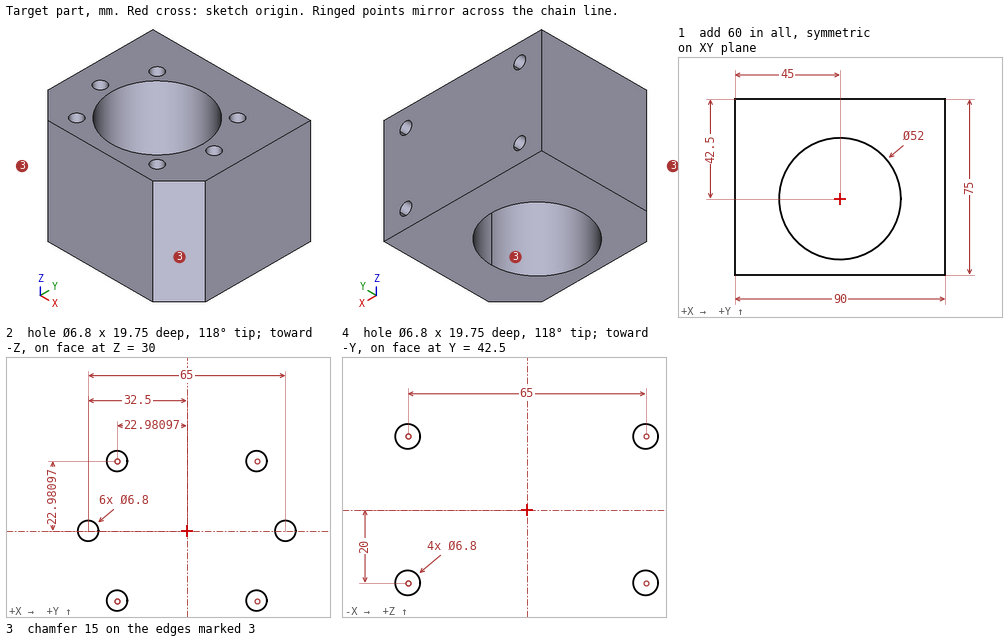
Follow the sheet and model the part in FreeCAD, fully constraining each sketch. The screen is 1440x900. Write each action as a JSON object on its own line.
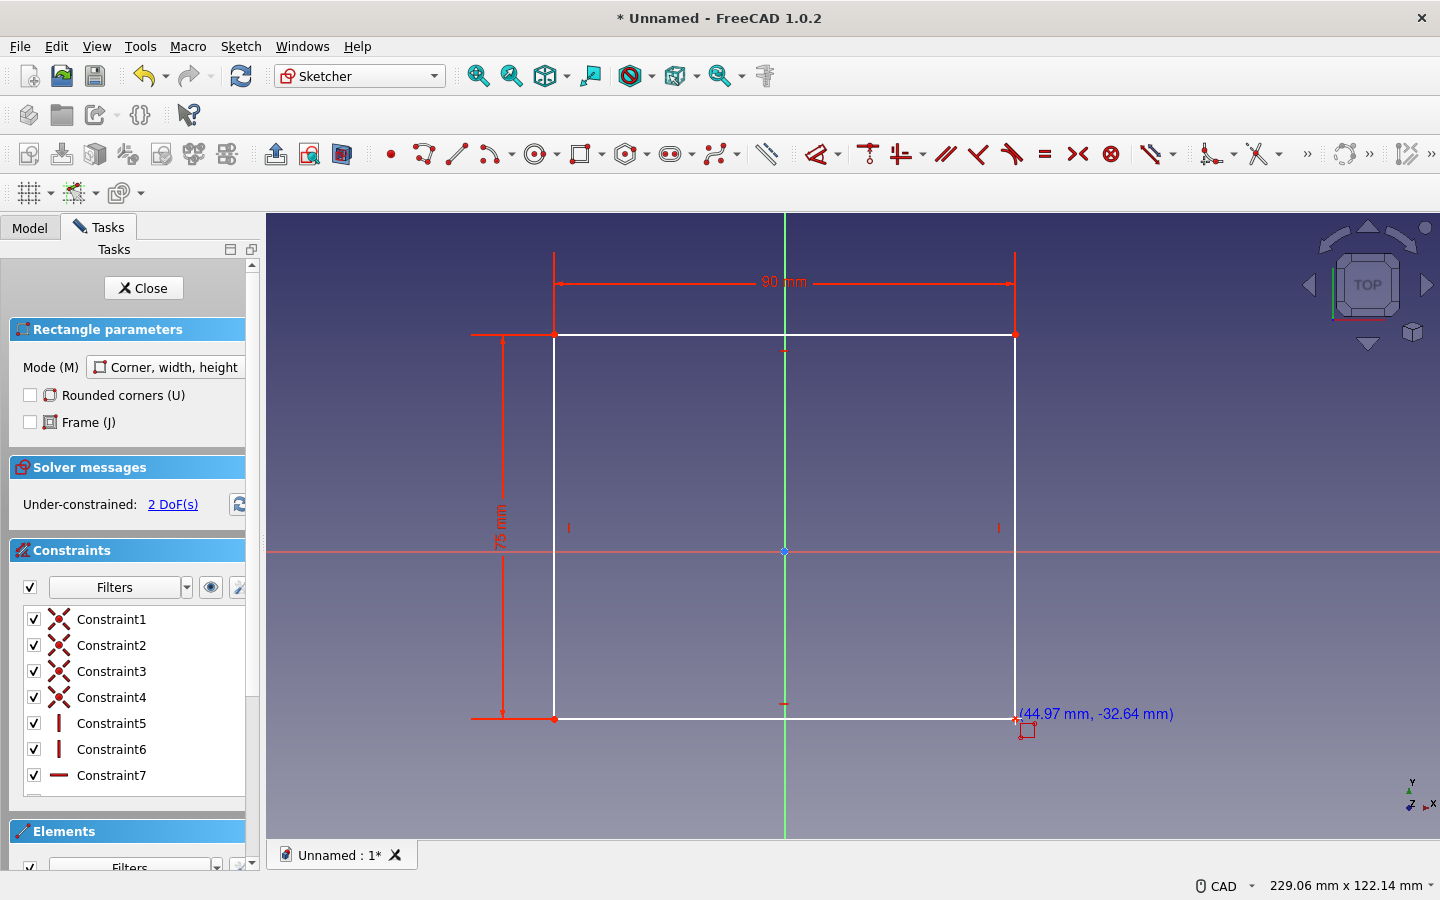
{"action": "key", "text": "g c"}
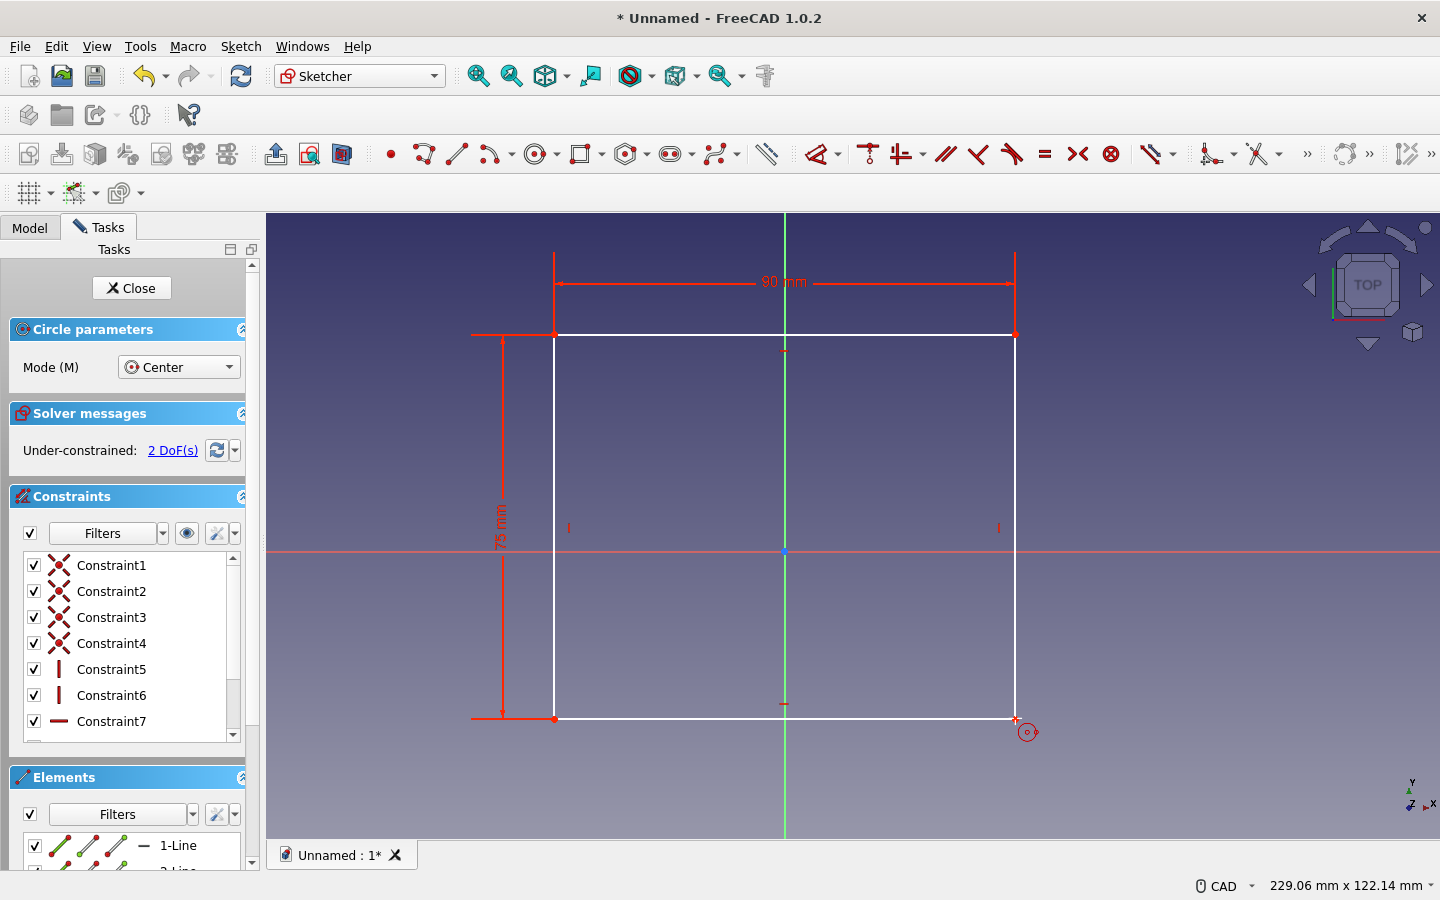
{"action": "left_click", "coordinate": [785, 552]}
{"action": "mouse_move", "coordinate": [879, 457]}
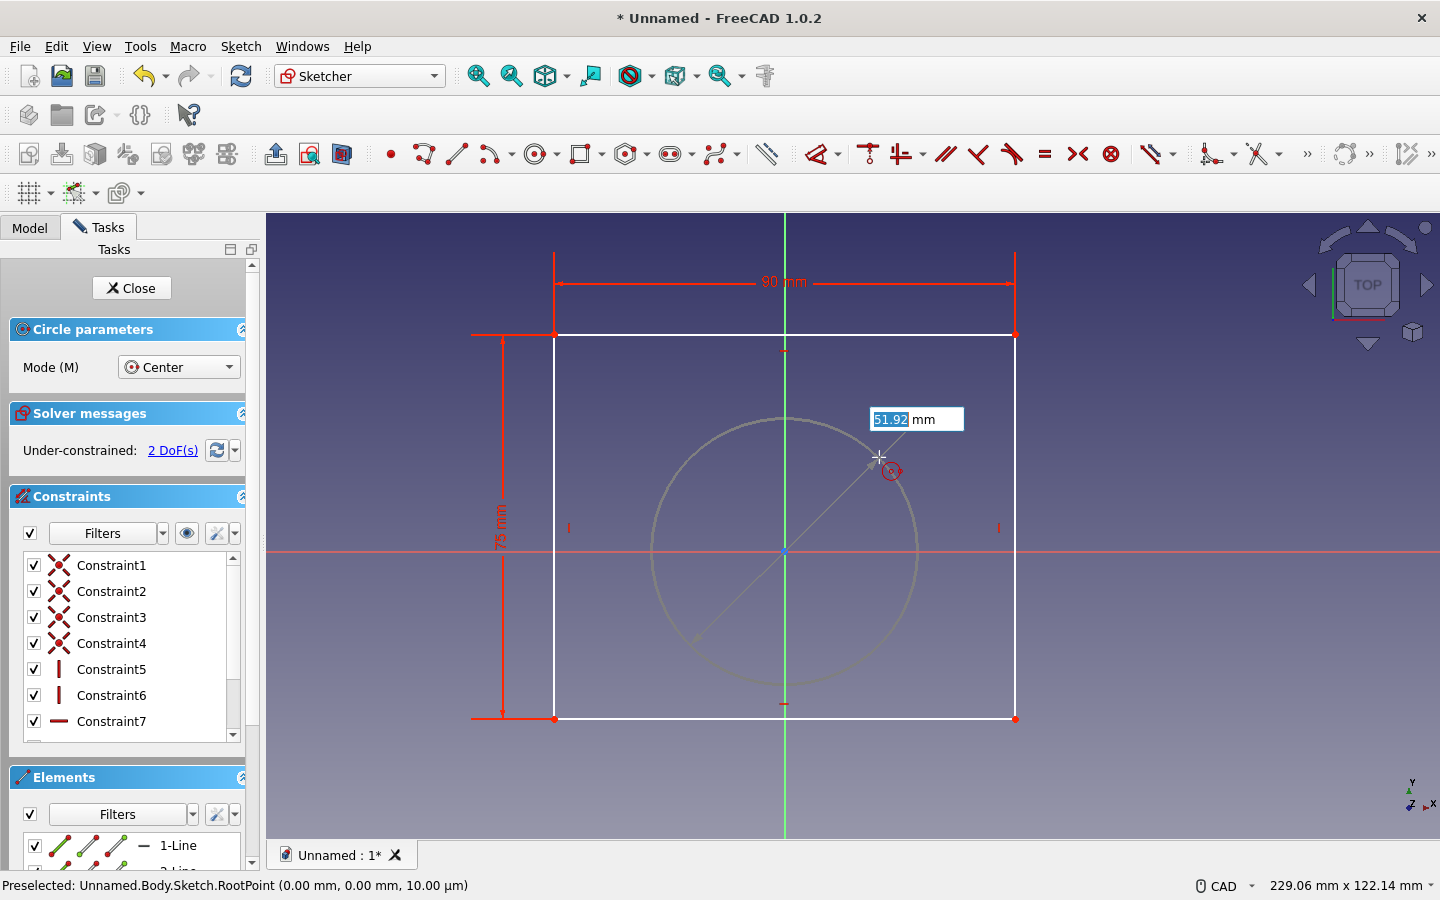
{"action": "type", "text": "52"}
{"action": "key", "text": "Return"}
{"action": "key", "text": "Escape"}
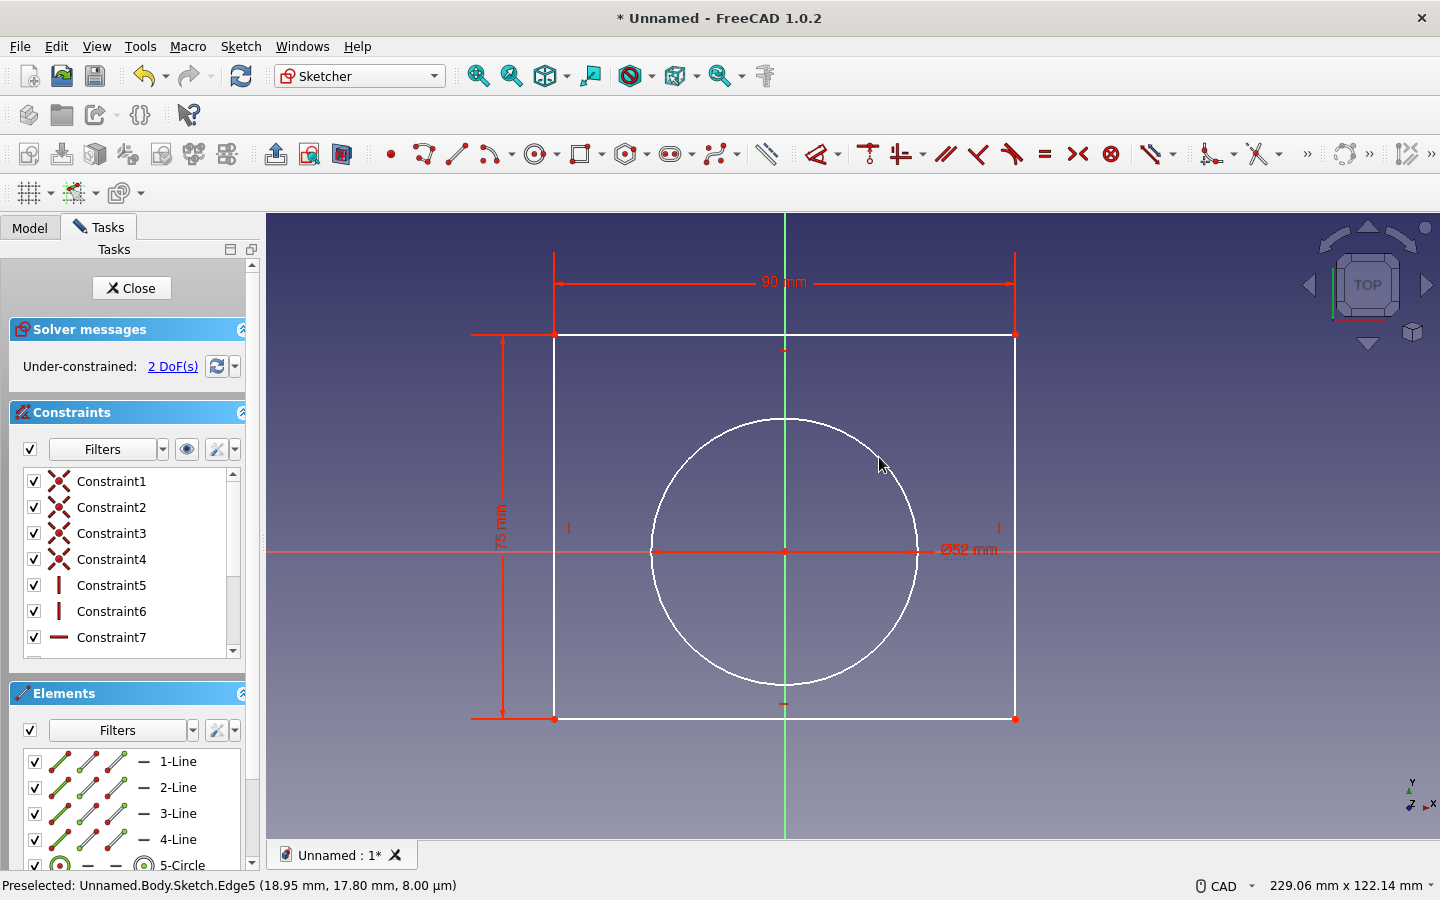
{"action": "left_click", "coordinate": [816, 154]}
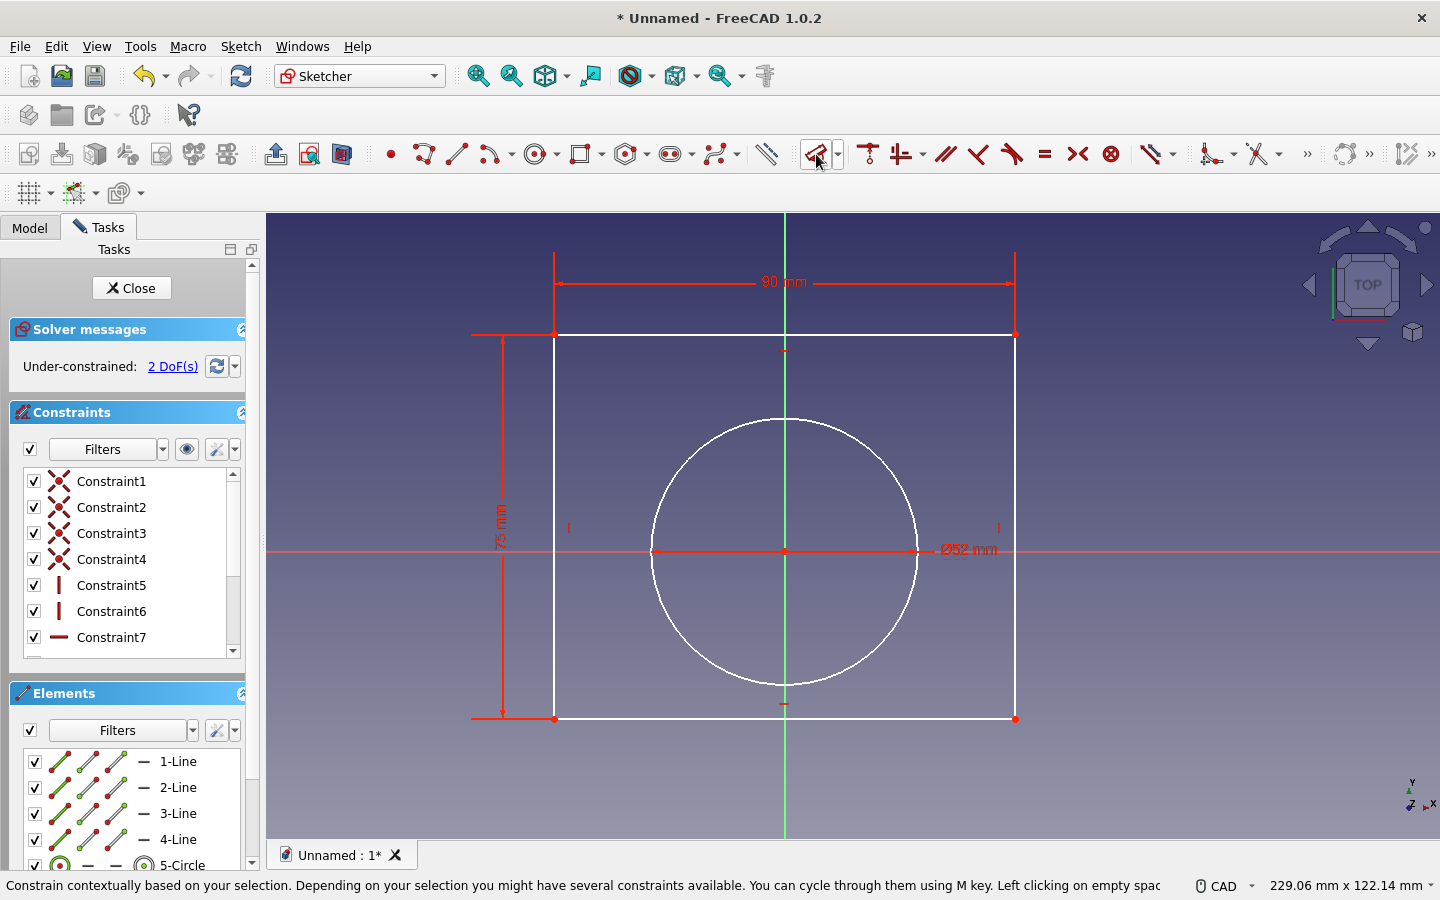
{"action": "left_click", "coordinate": [554, 335]}
{"action": "left_click", "coordinate": [669, 301]}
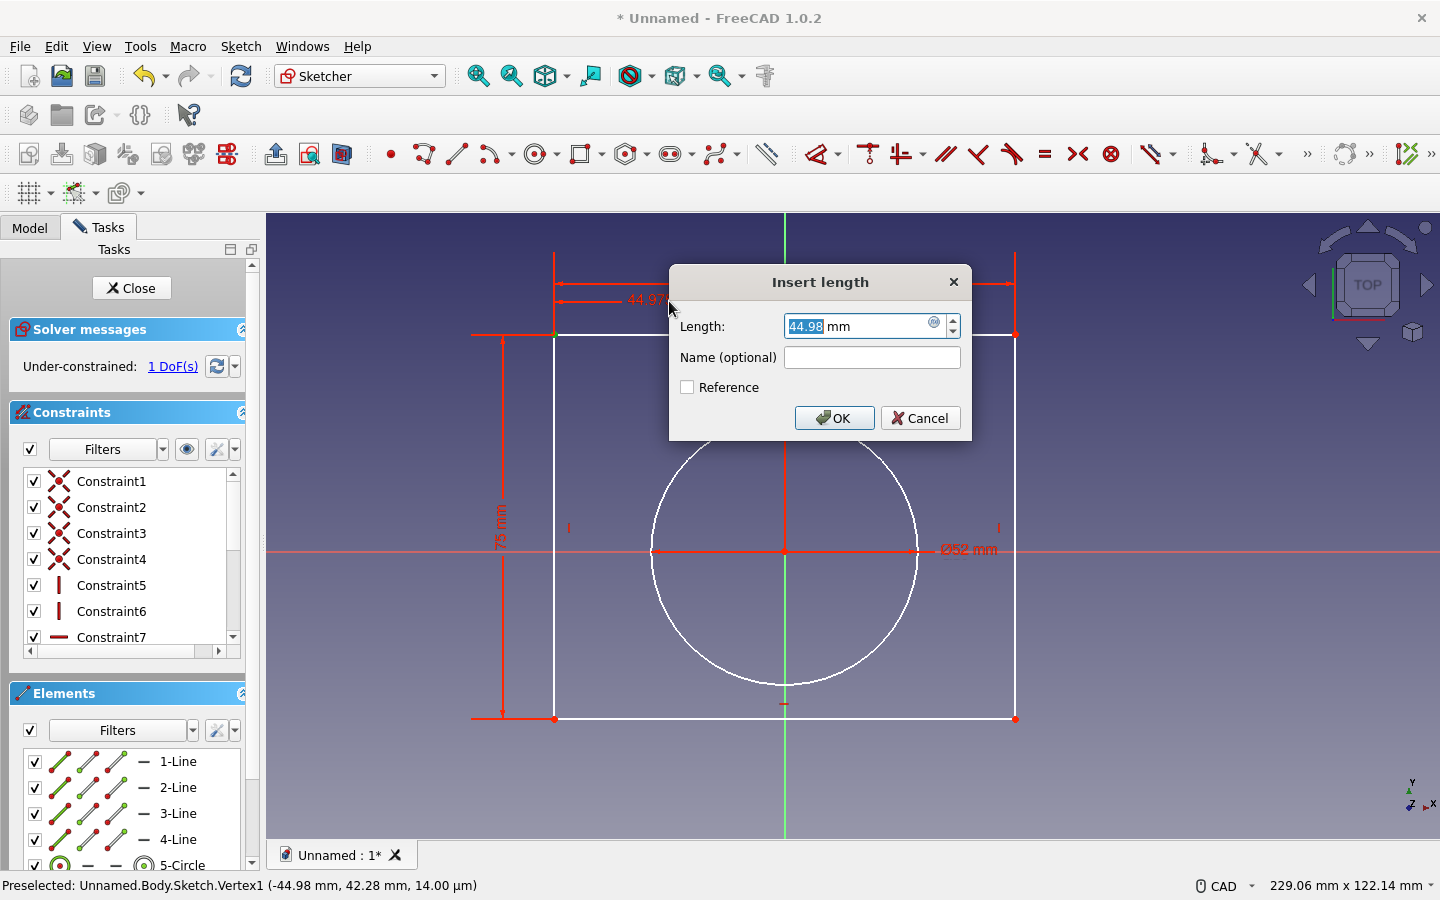
{"action": "type", "text": "45"}
{"action": "key", "text": "Return"}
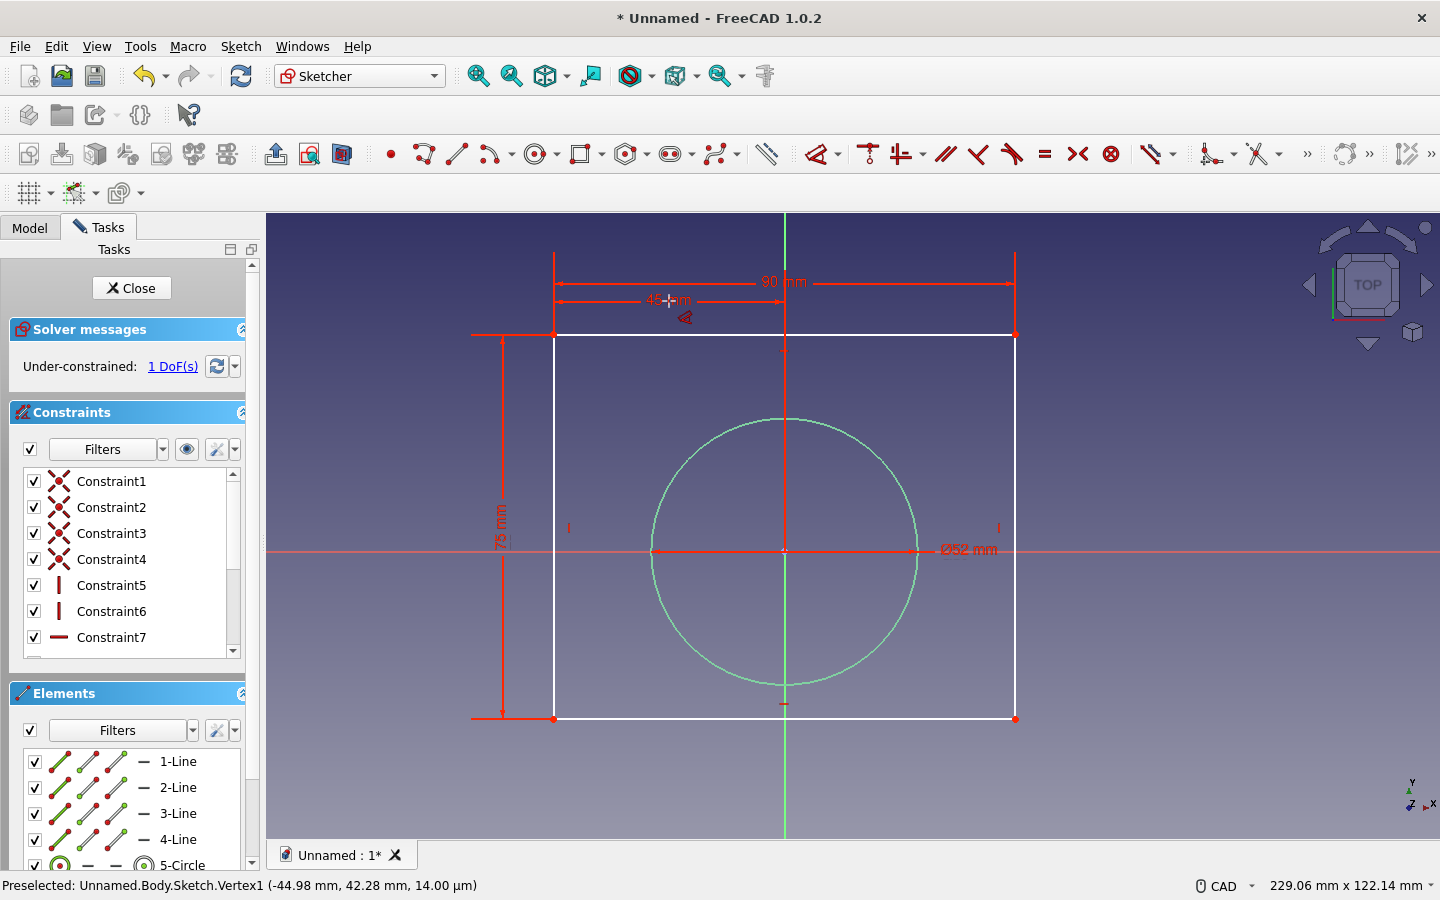
{"action": "left_click", "coordinate": [554, 335]}
{"action": "left_click", "coordinate": [520, 443]}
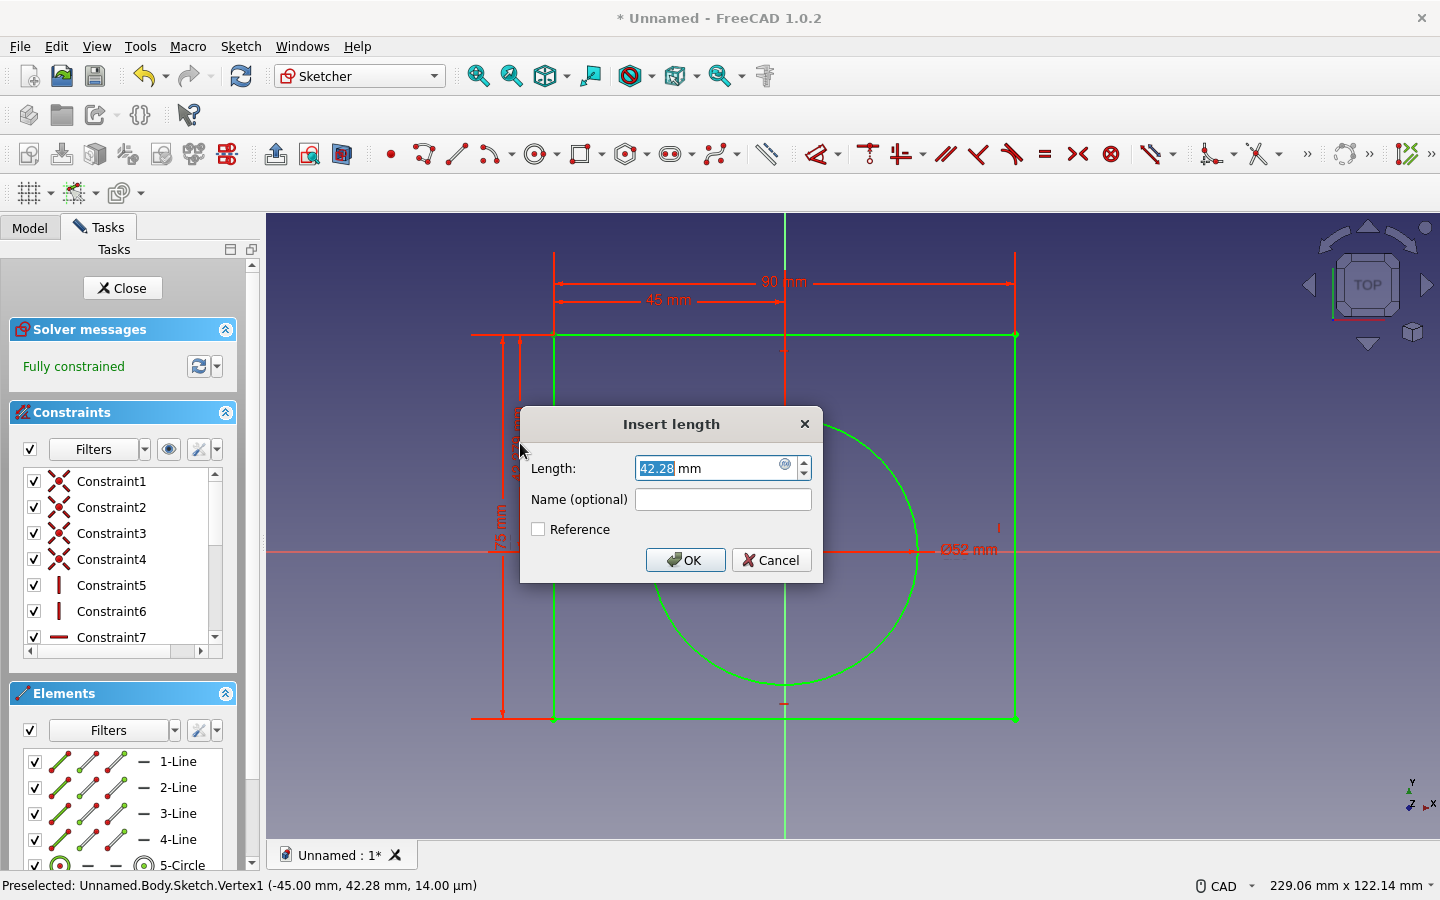
{"action": "type", "text": "42.5"}
{"action": "key", "text": "Return"}
{"action": "key", "text": "Escape"}